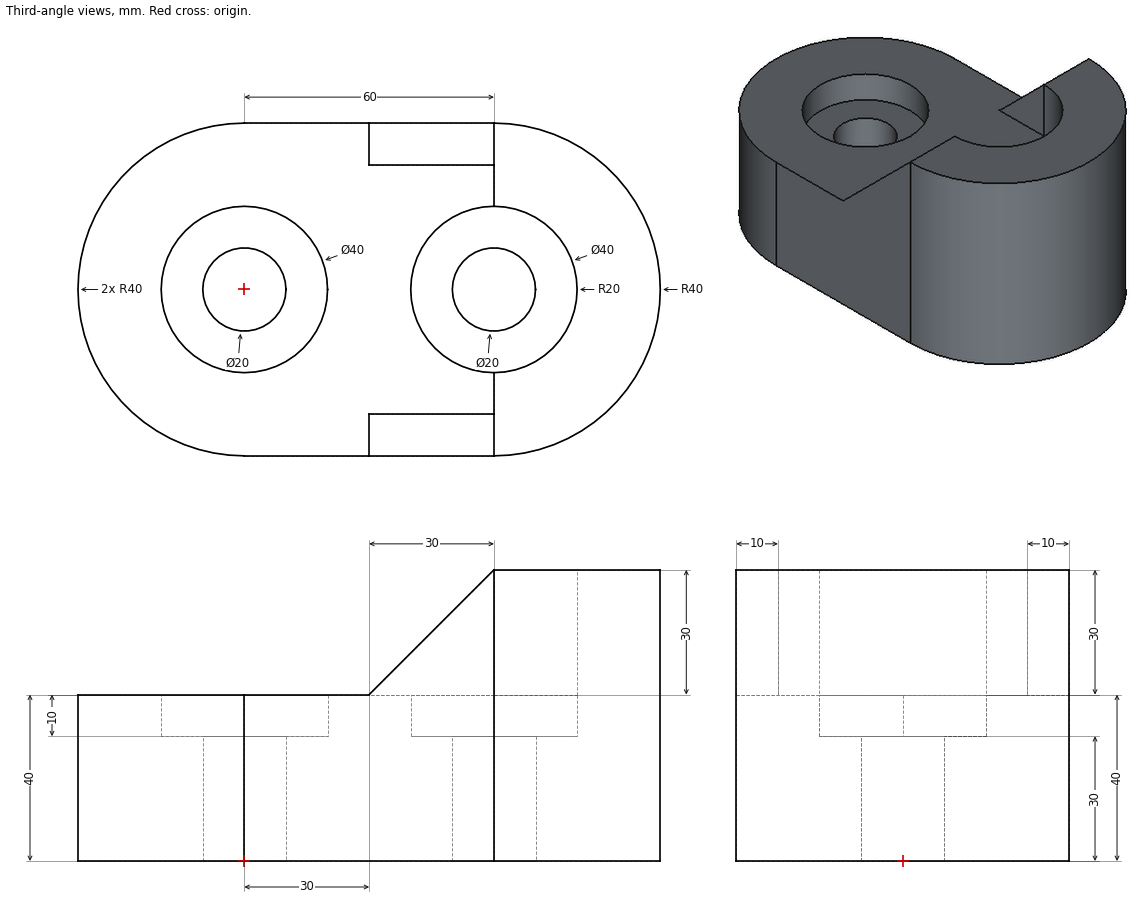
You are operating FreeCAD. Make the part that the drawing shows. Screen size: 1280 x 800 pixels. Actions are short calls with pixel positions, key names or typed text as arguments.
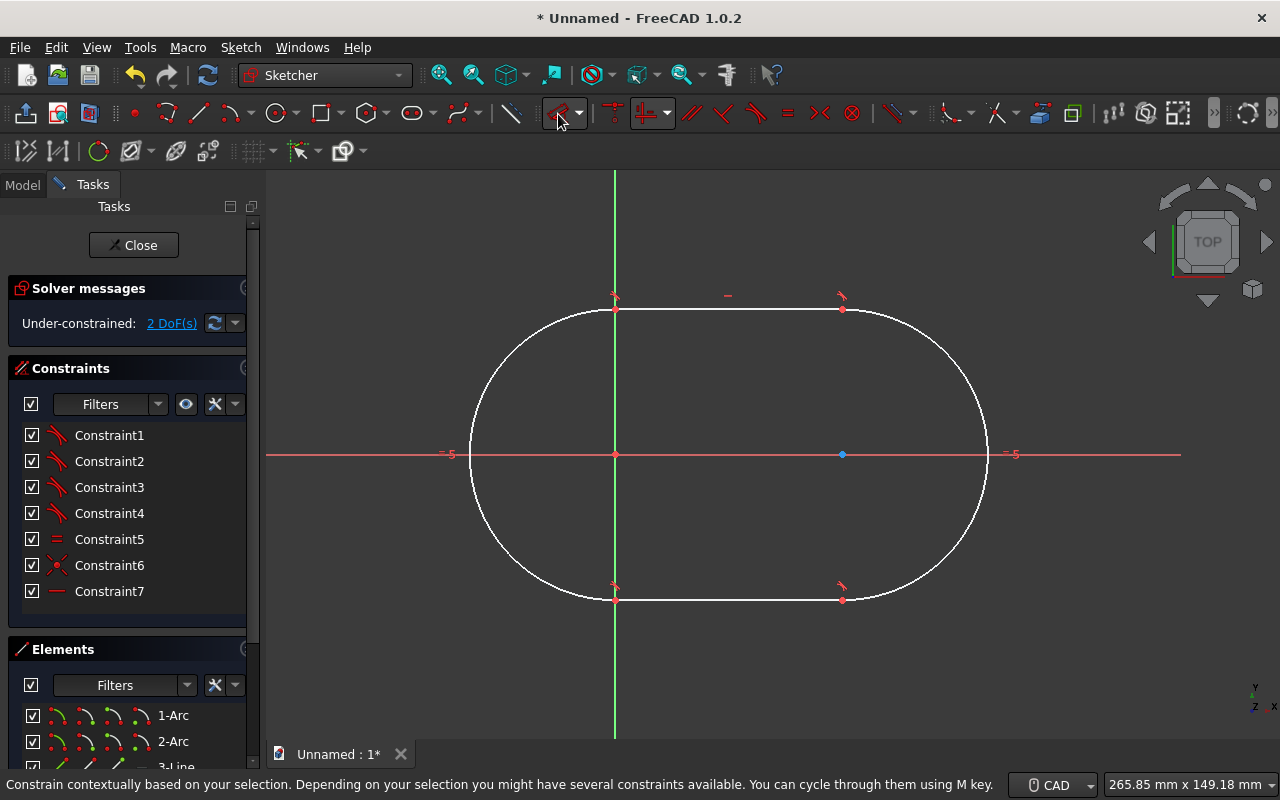
click(497, 369)
click(471, 350)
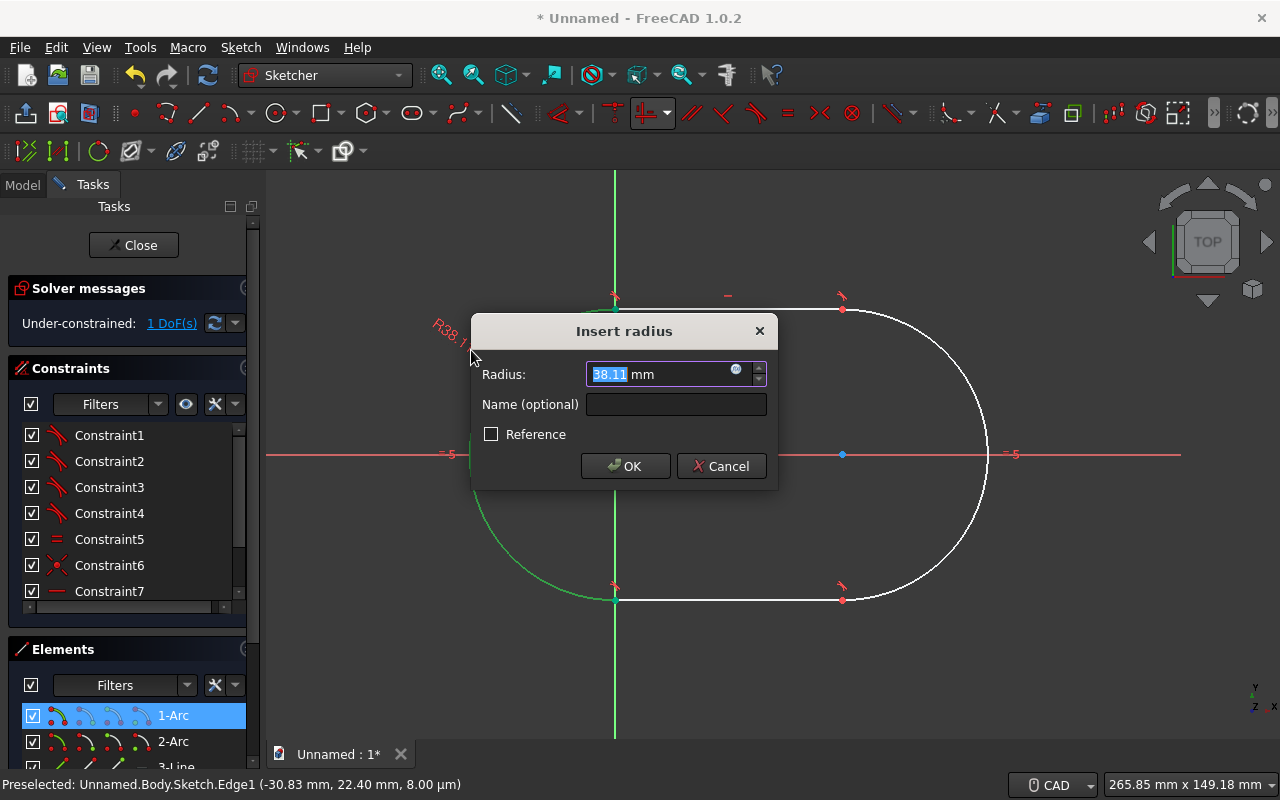
text(40)
key(Return)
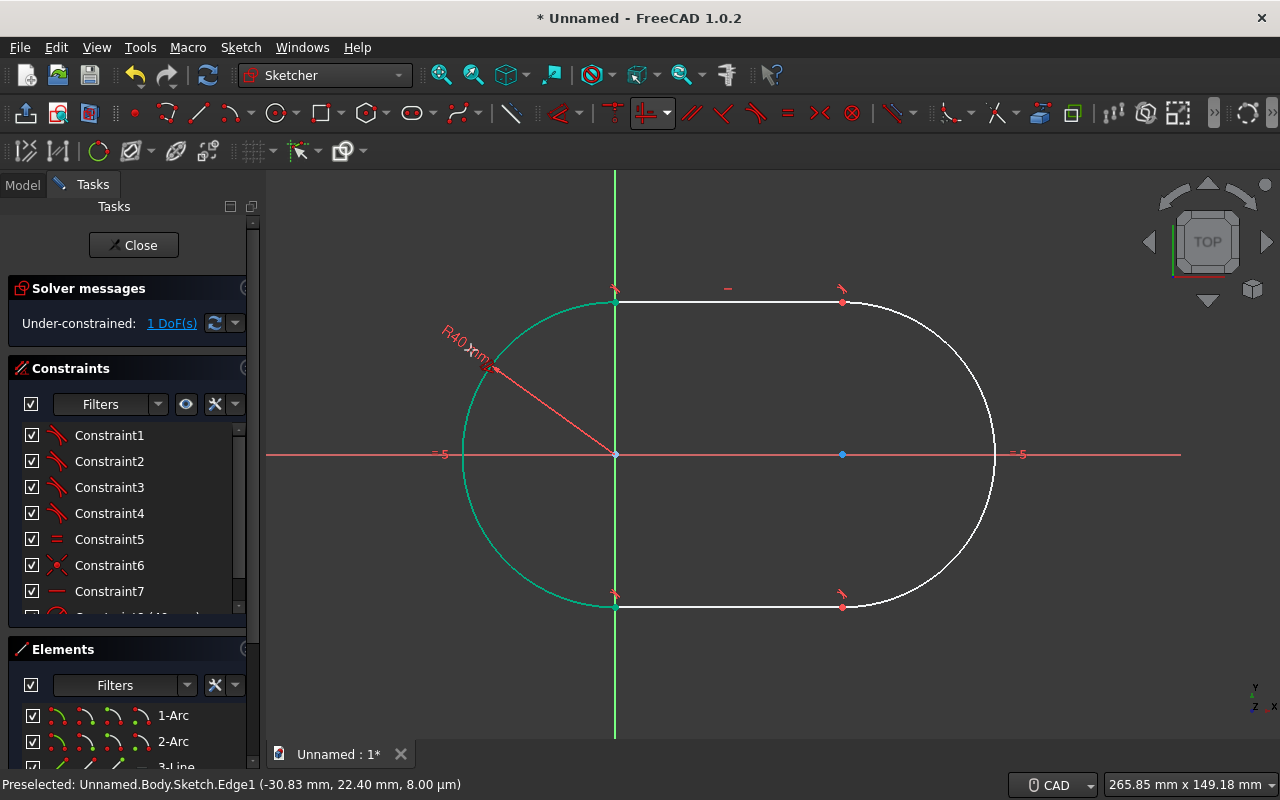
click(683, 302)
click(729, 268)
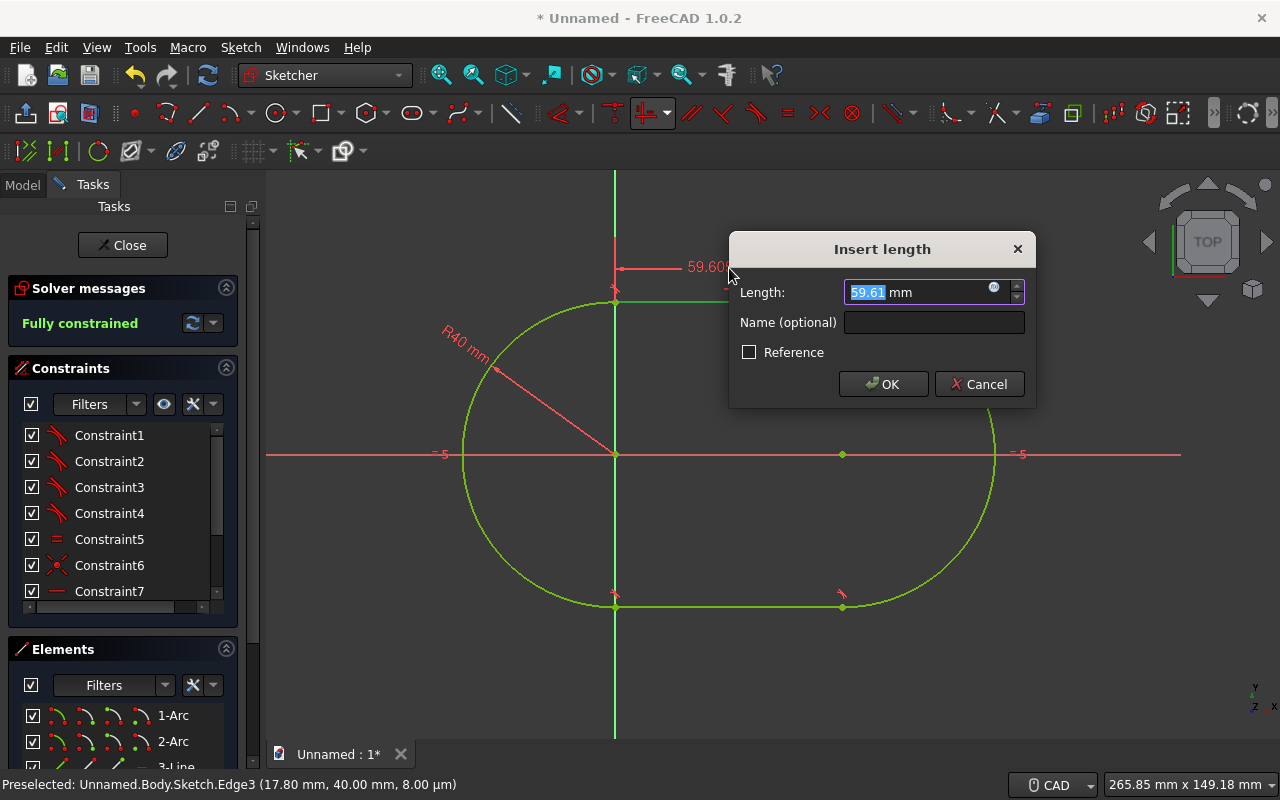
text(60)
key(Return)
key(Escape)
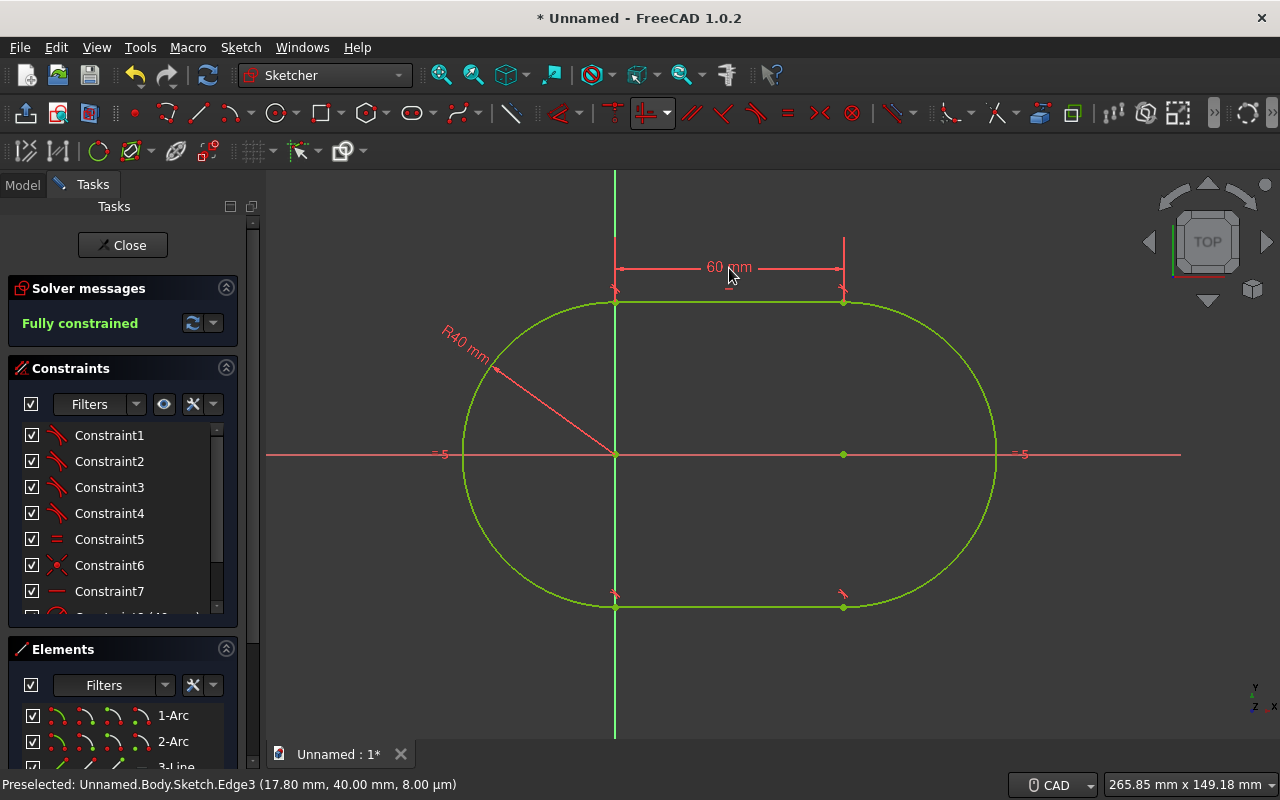
click(123, 245)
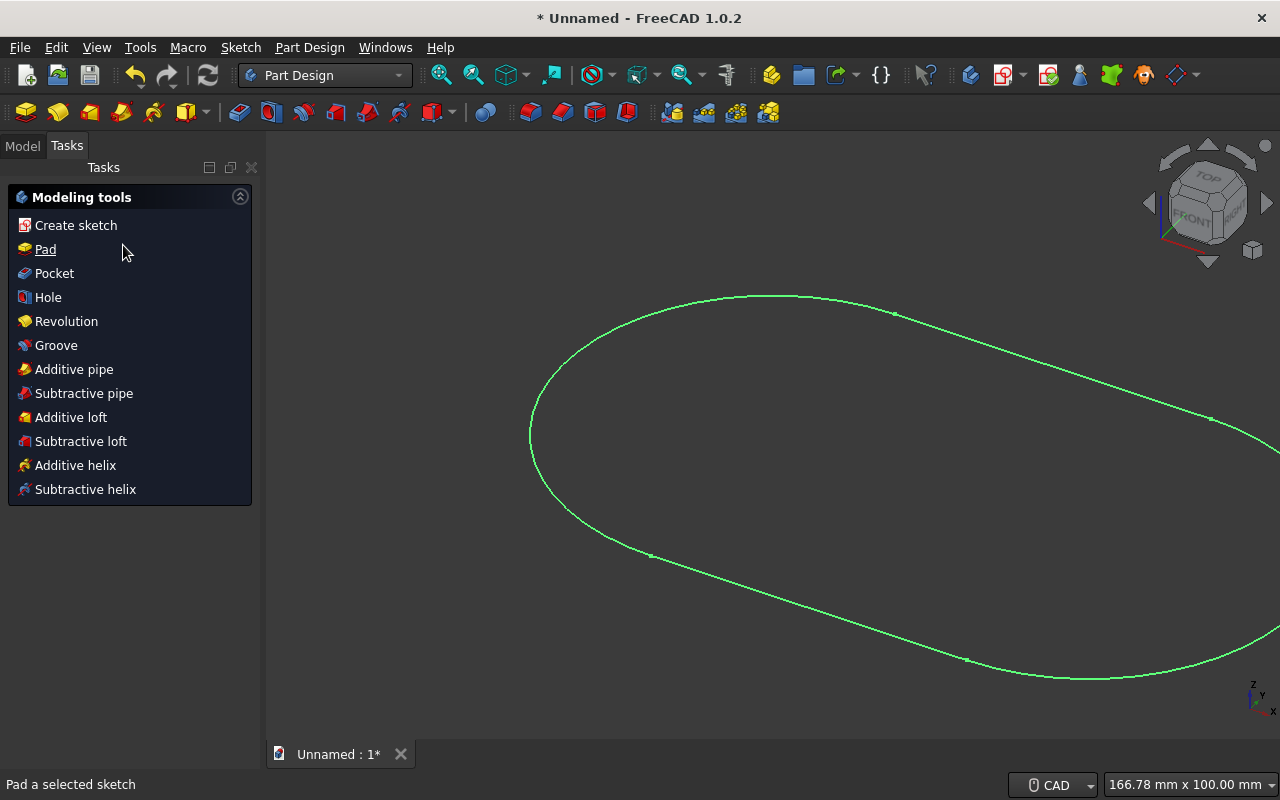
click(26, 112)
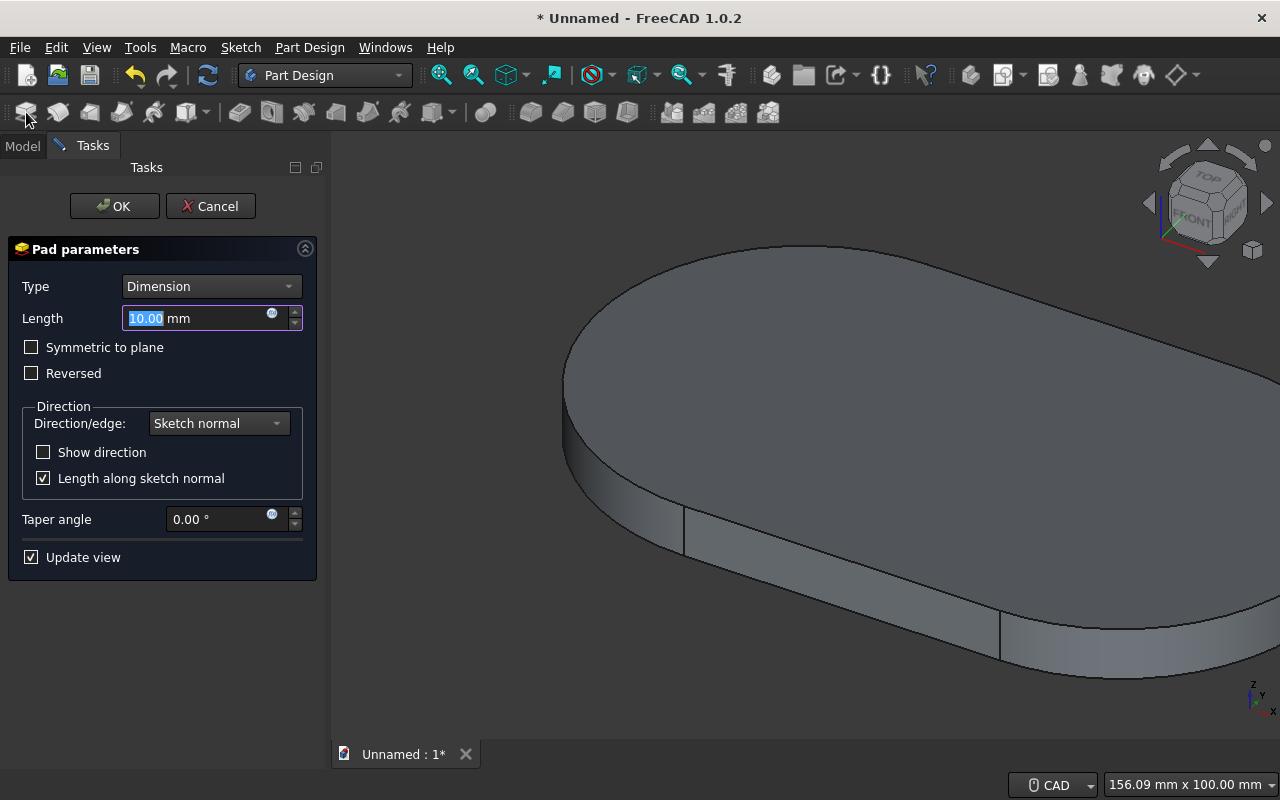
text(40)
key(Tab)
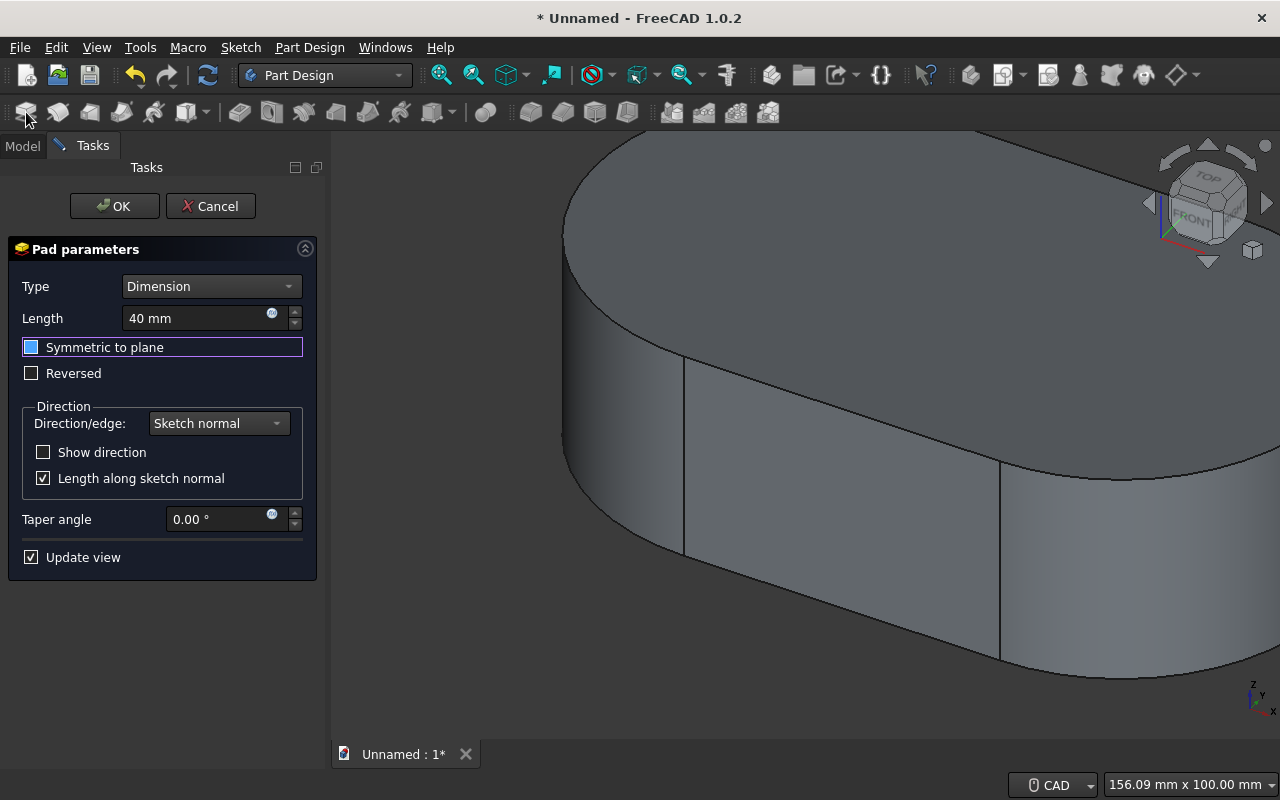
click(115, 206)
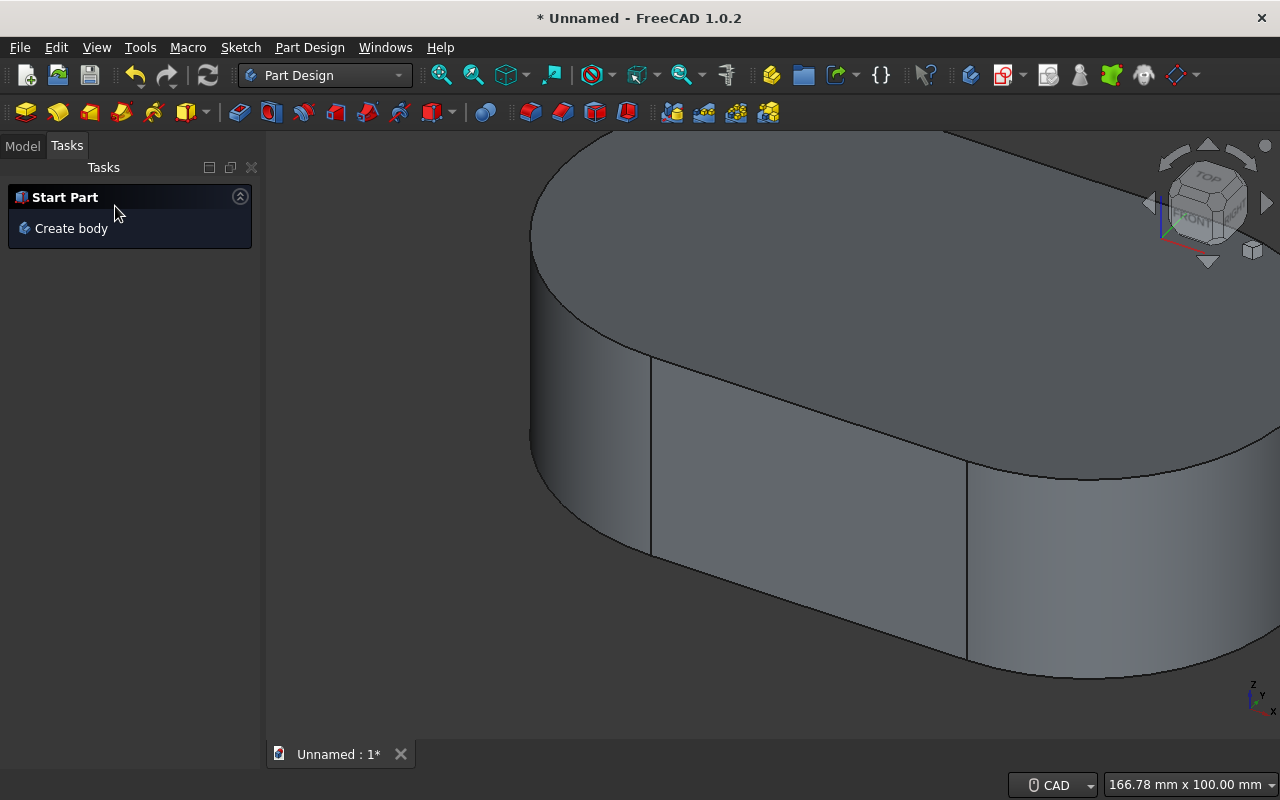
click(442, 76)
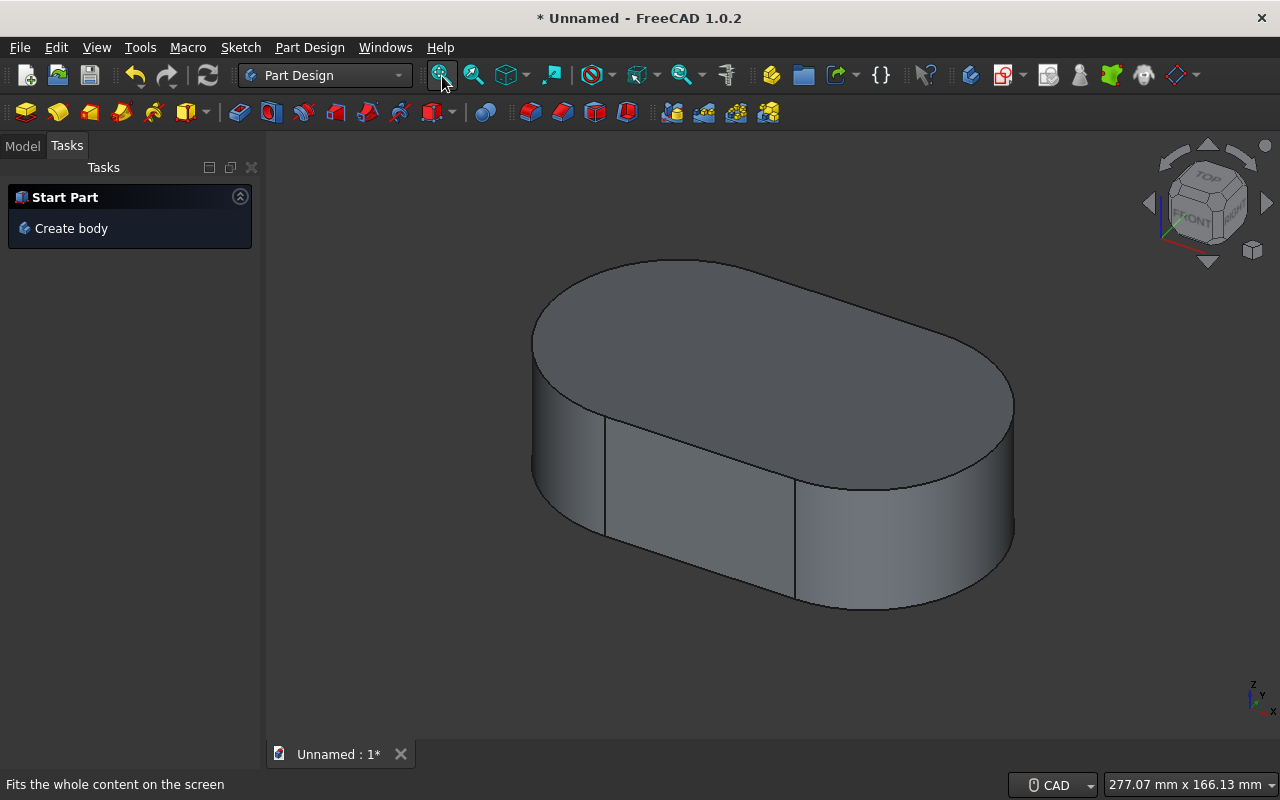
click(836, 395)